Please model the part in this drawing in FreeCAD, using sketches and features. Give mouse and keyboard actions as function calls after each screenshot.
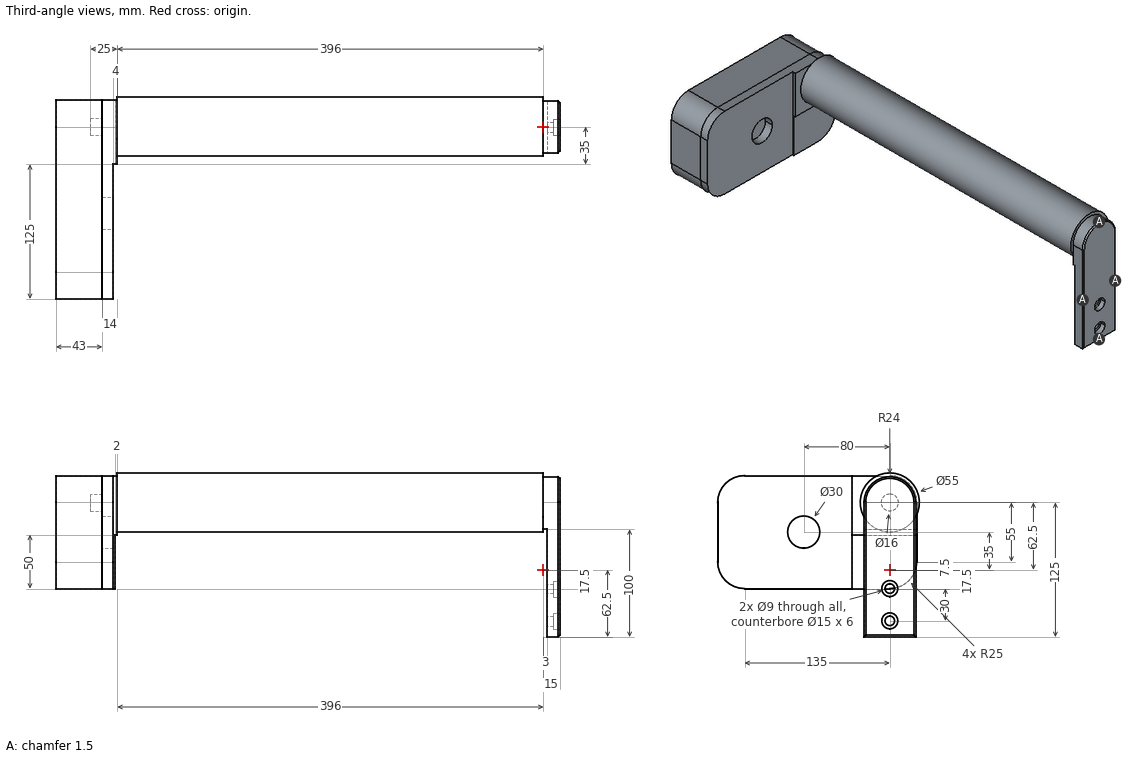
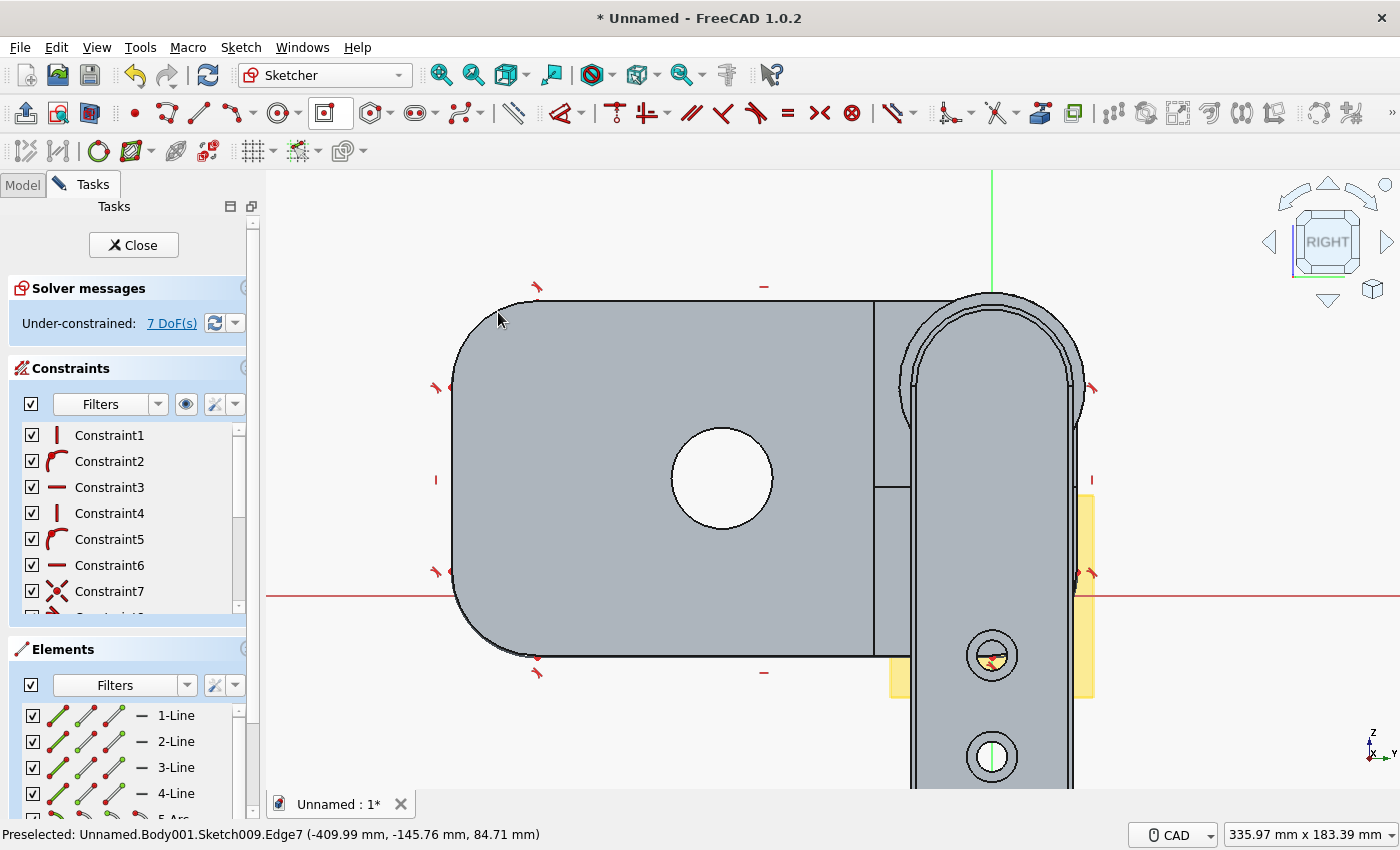
click(674, 302)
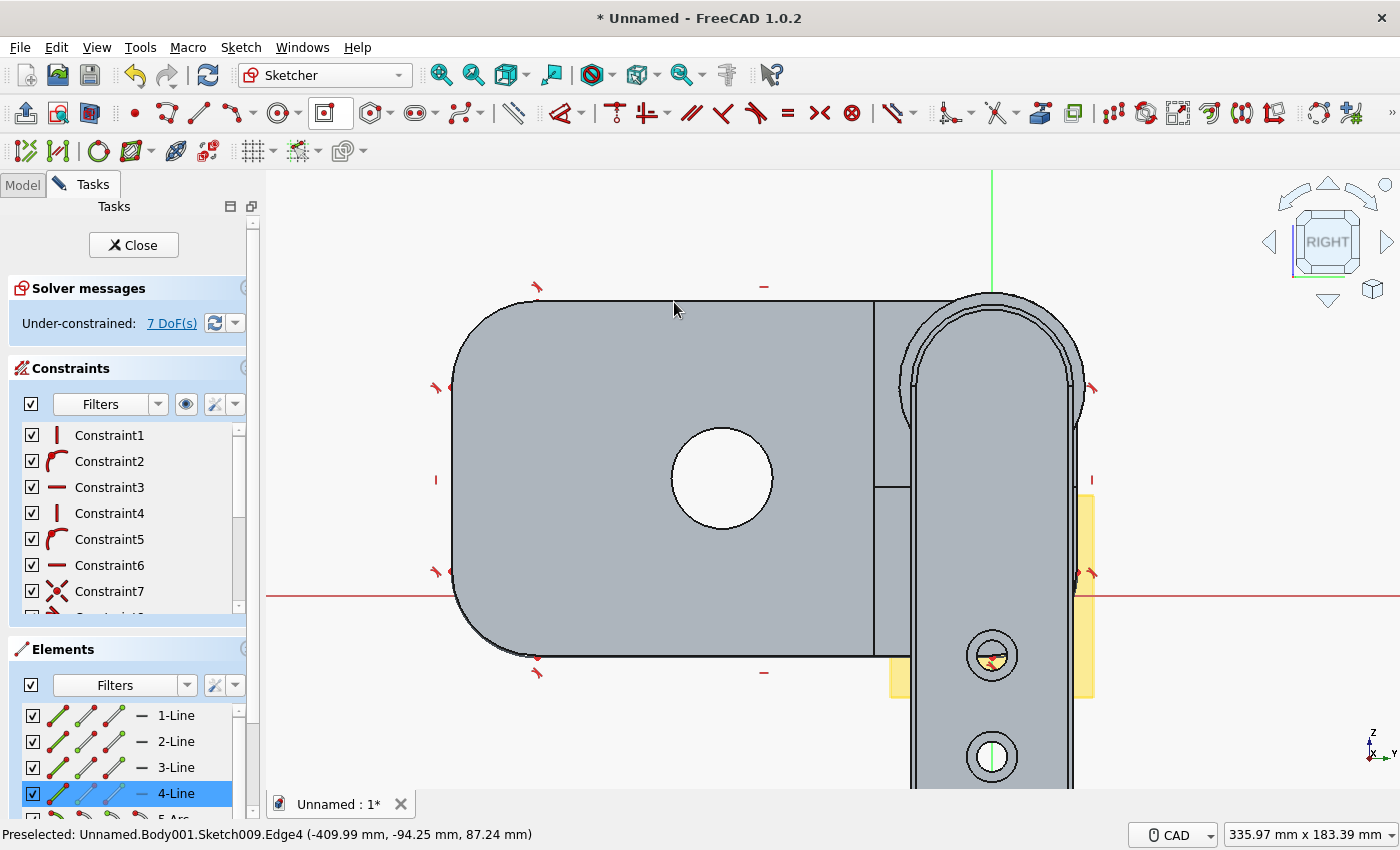
click(1068, 349)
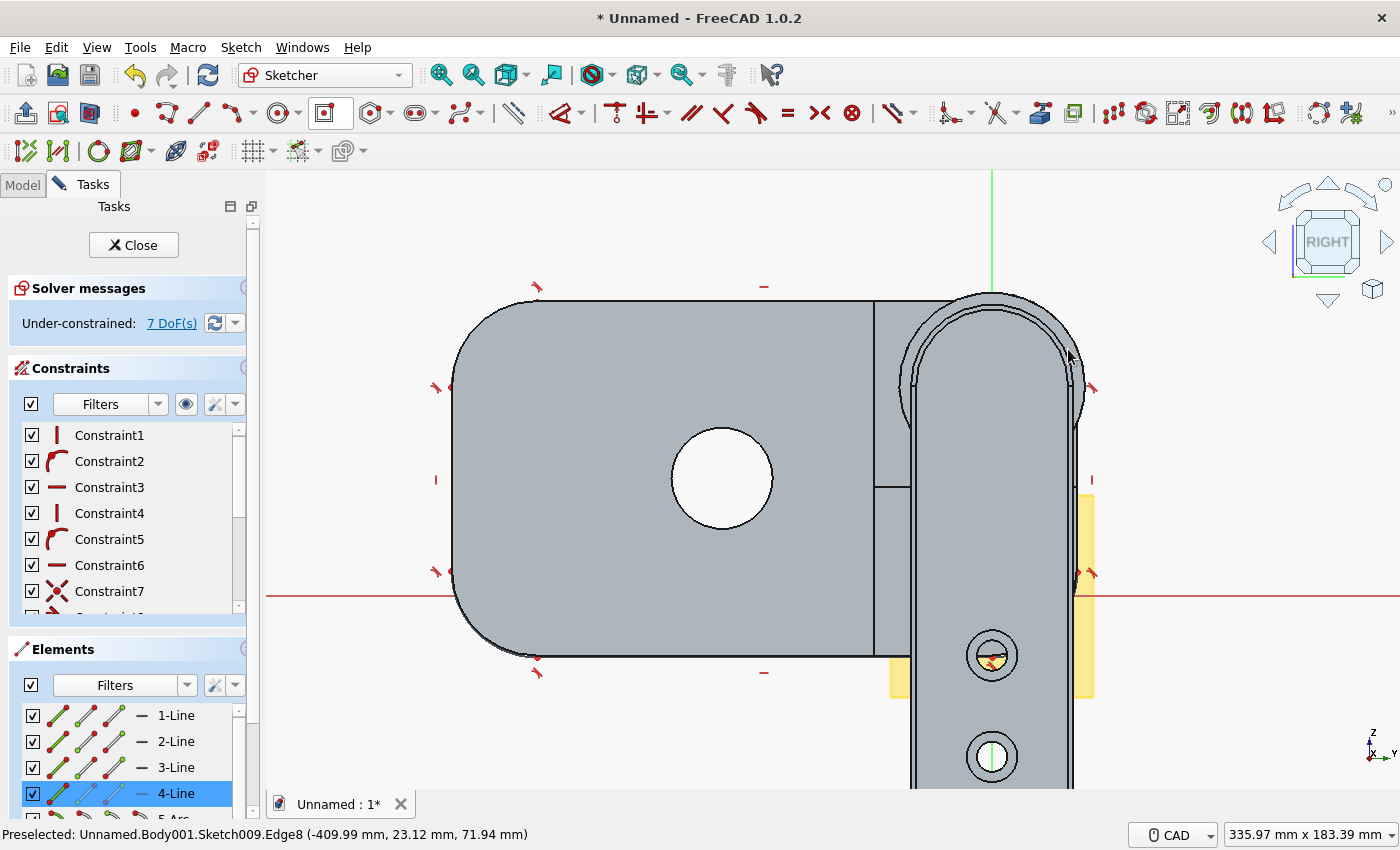
key(t)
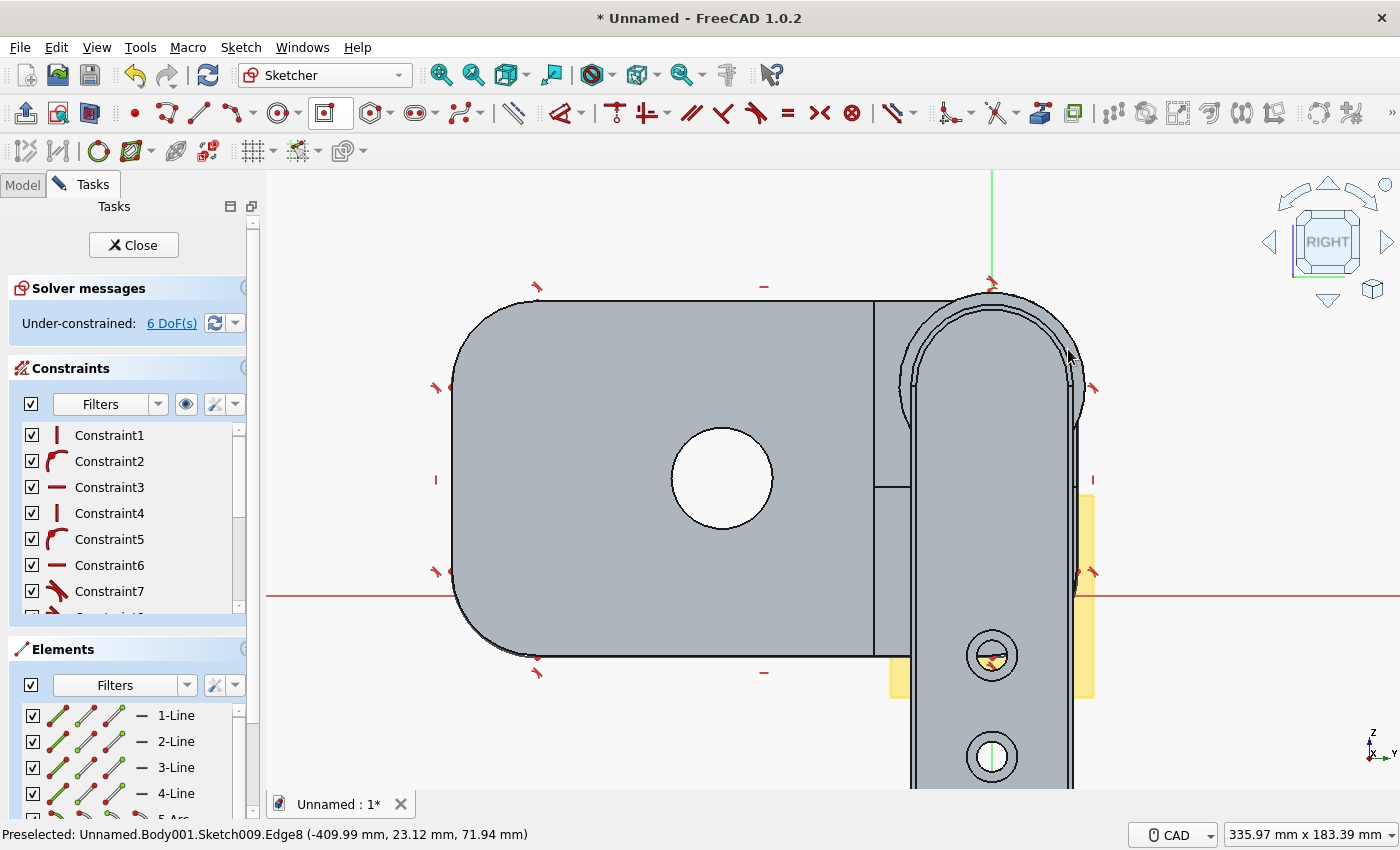
click(1031, 648)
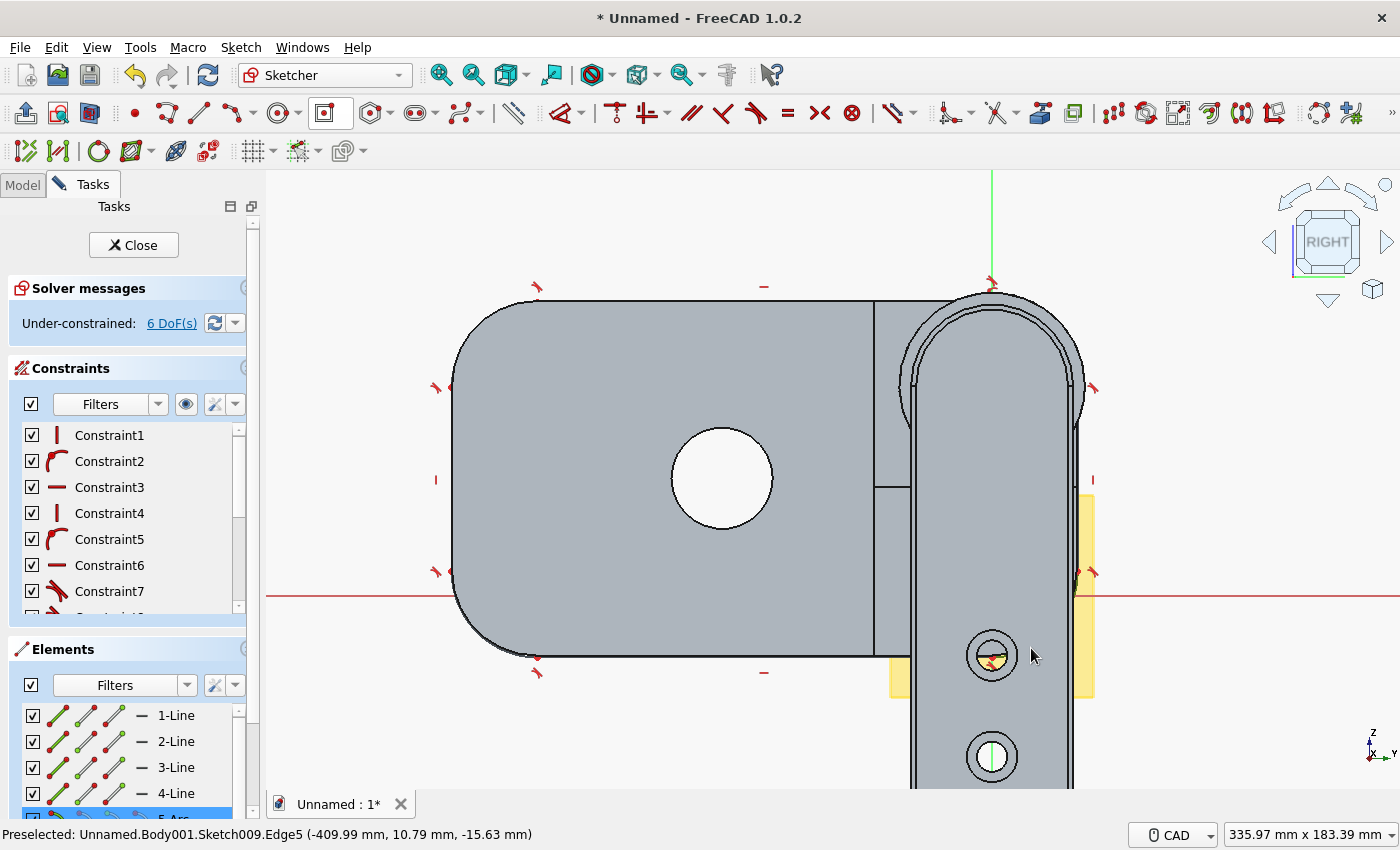
click(461, 611)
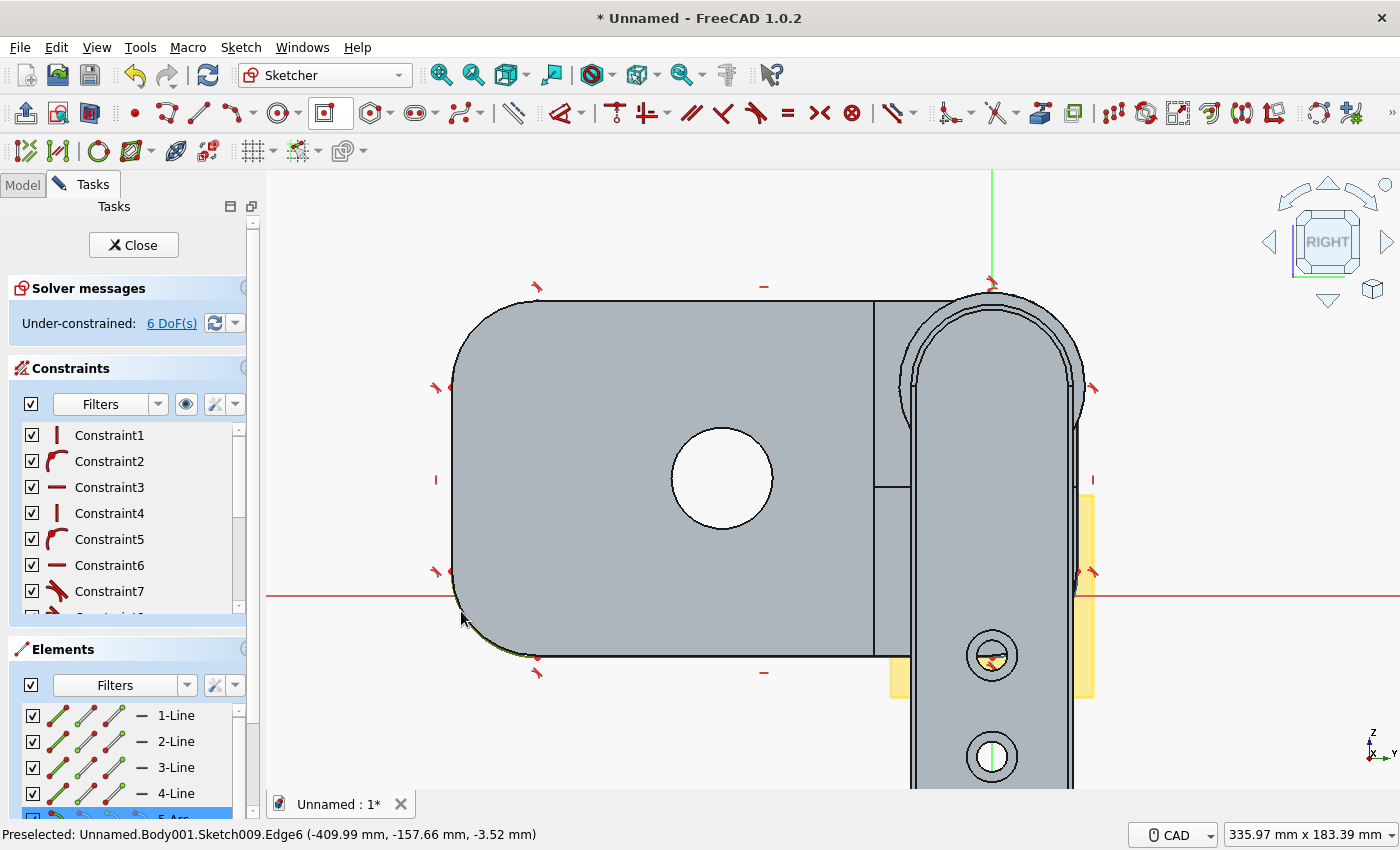
click(498, 311)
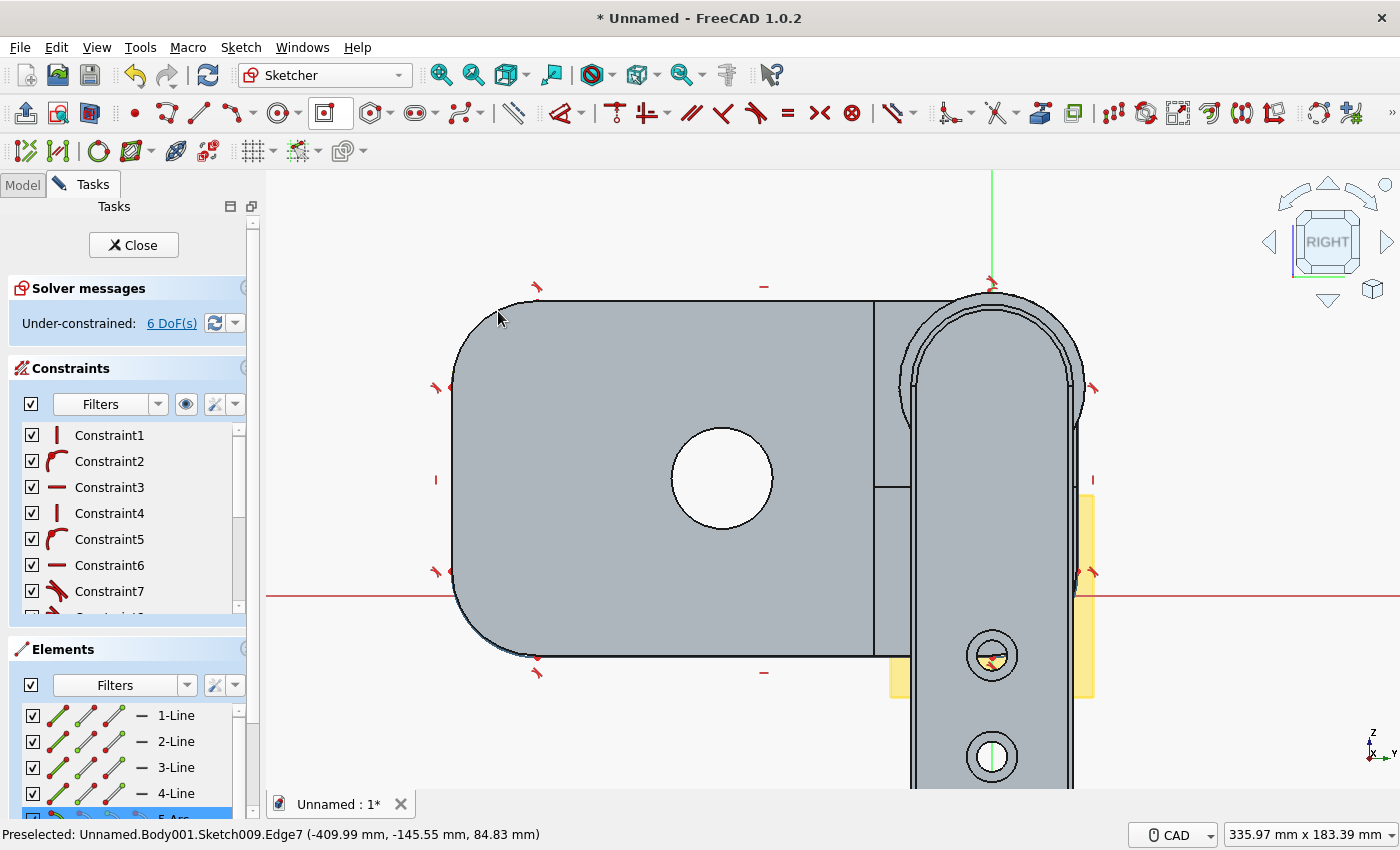
key(e)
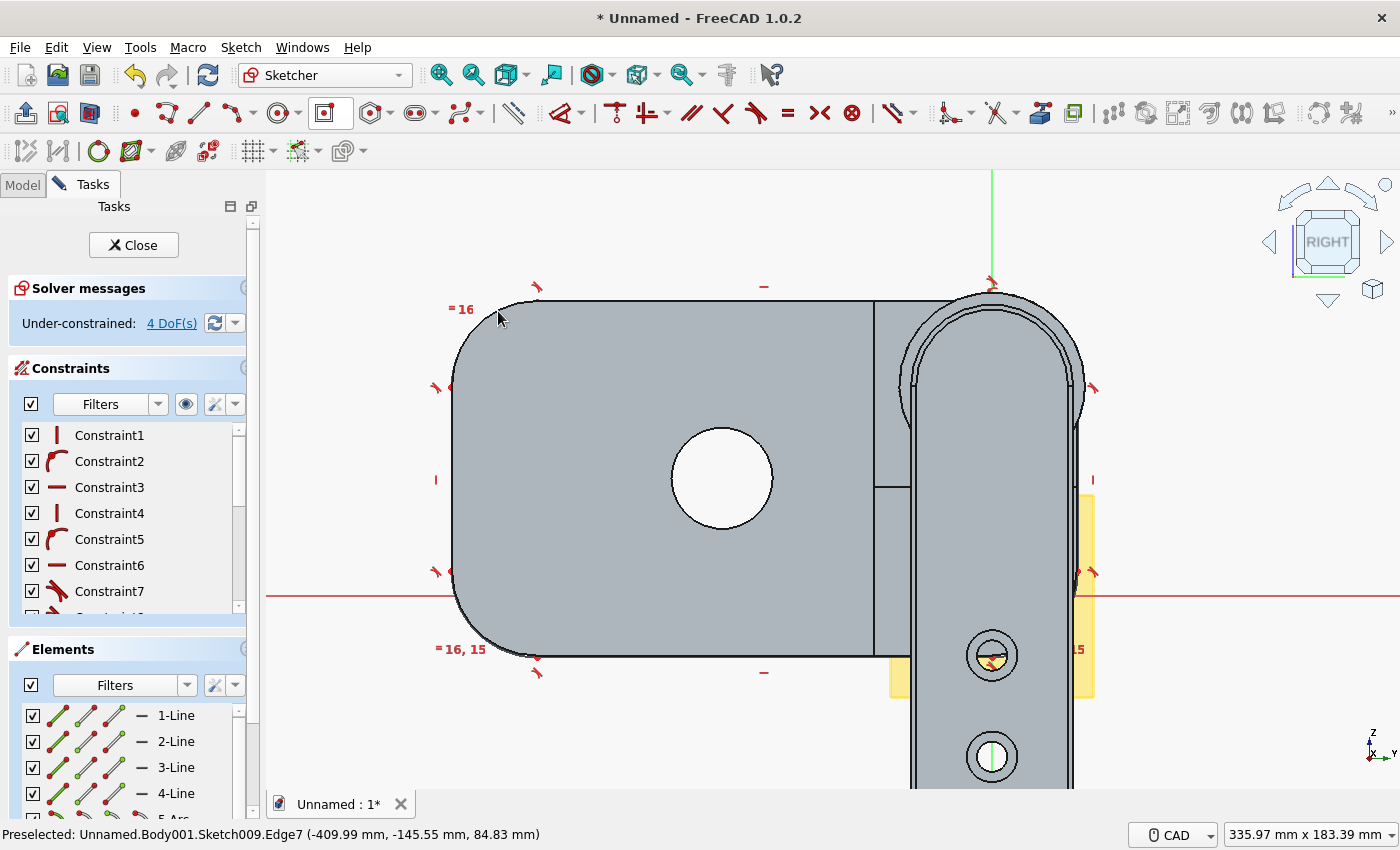
key(d)